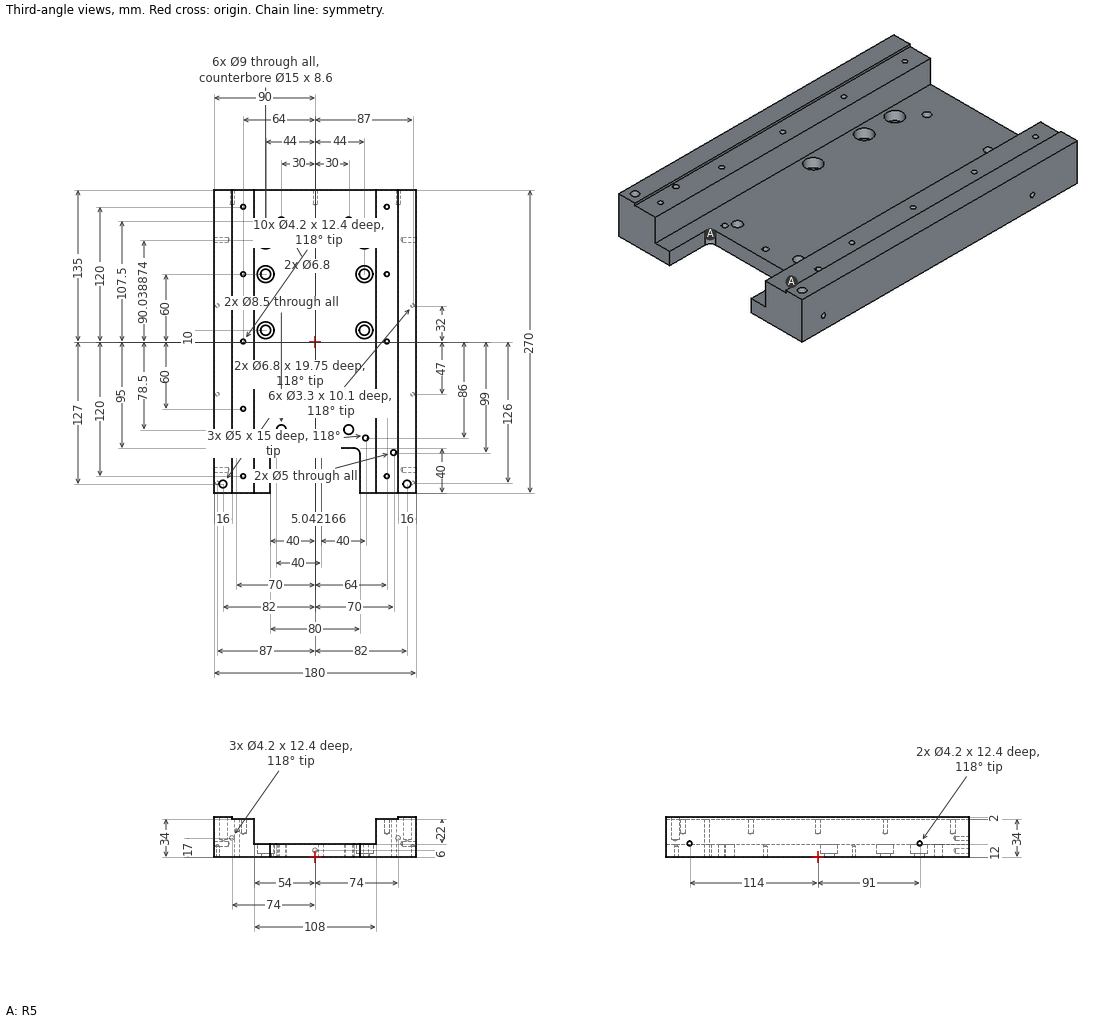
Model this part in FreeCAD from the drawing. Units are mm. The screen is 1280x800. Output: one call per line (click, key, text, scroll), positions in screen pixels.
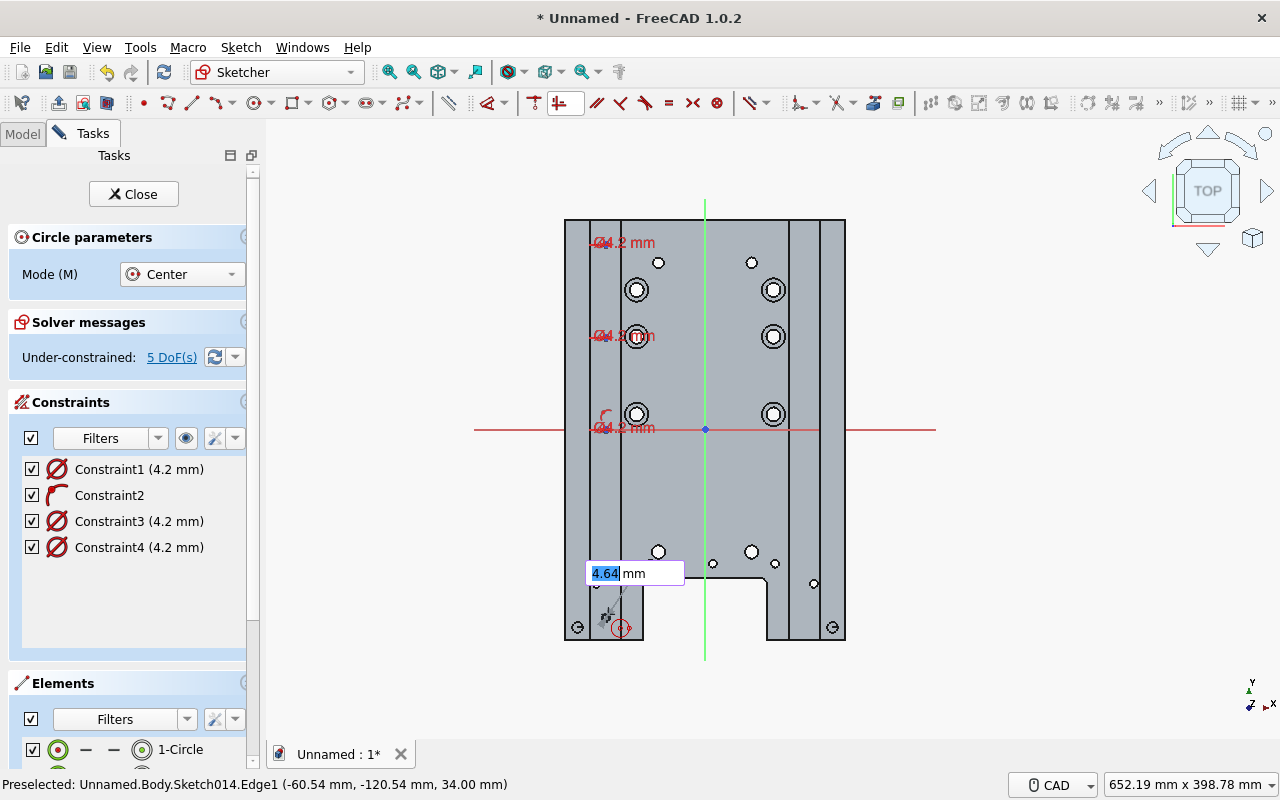
text(4.2)
key(Return)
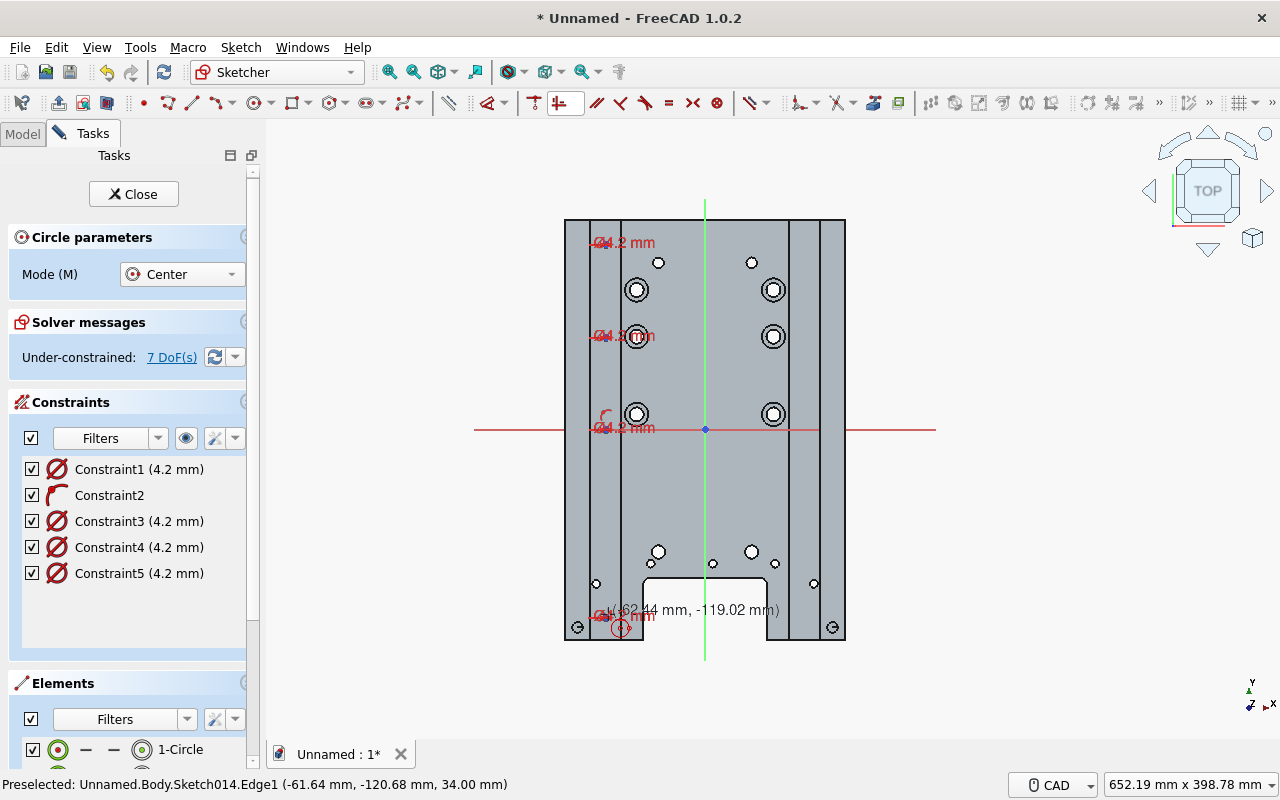
scroll(606, 523, up, 10)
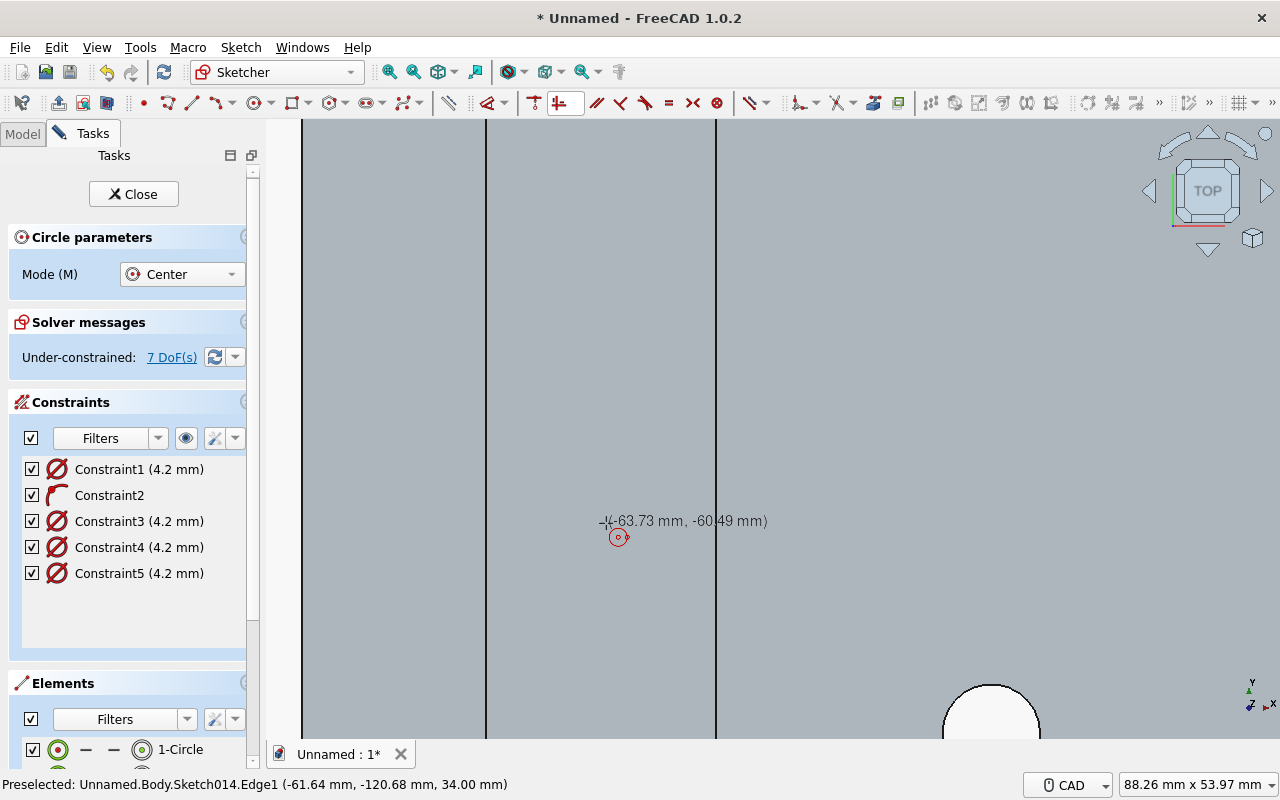
scroll(606, 523, down, 10)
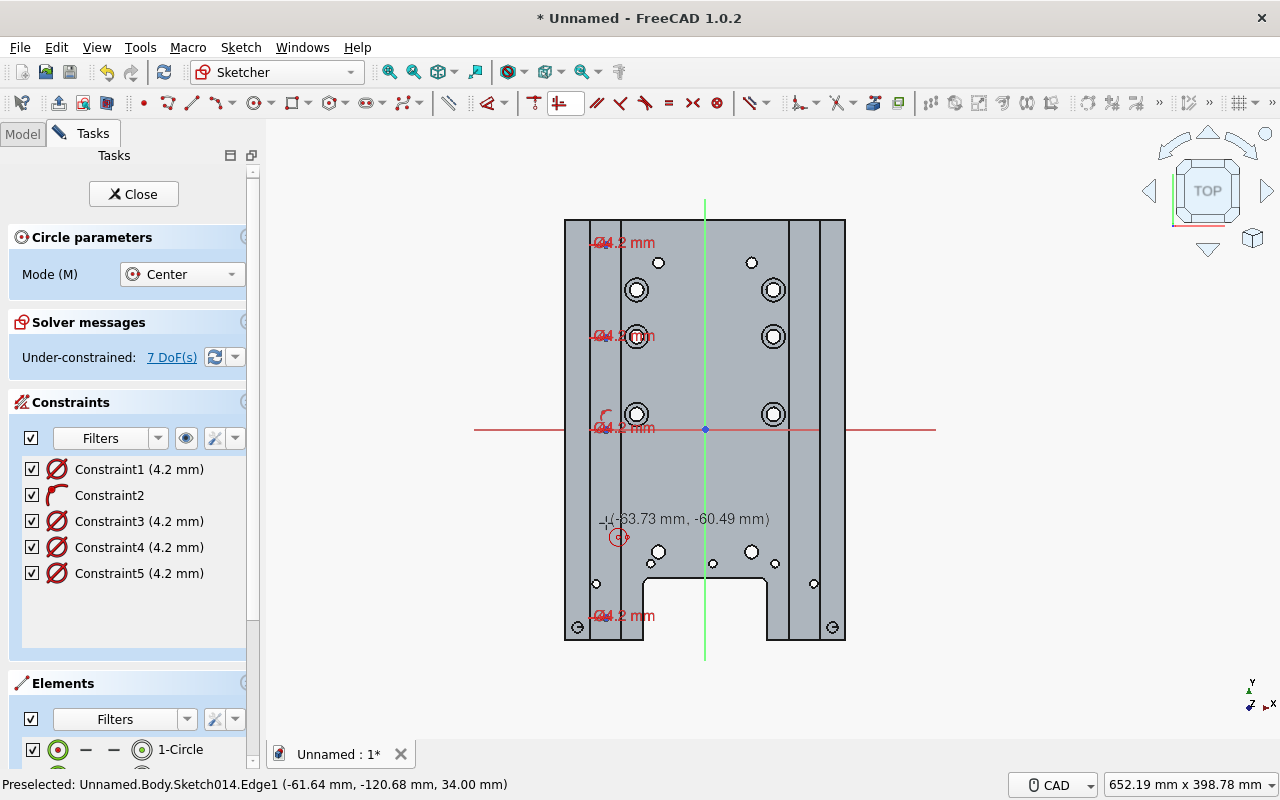
click(606, 523)
move(608, 521)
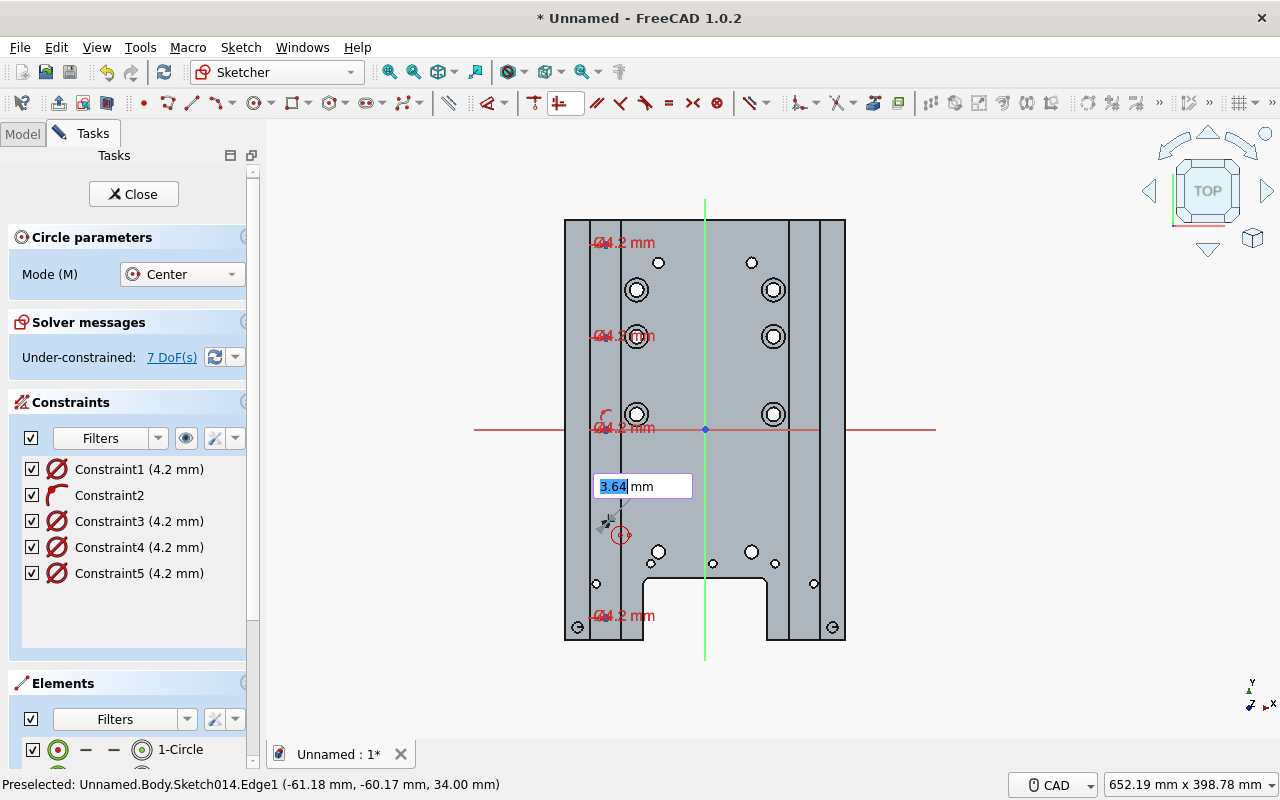
text(4.2)
key(Return)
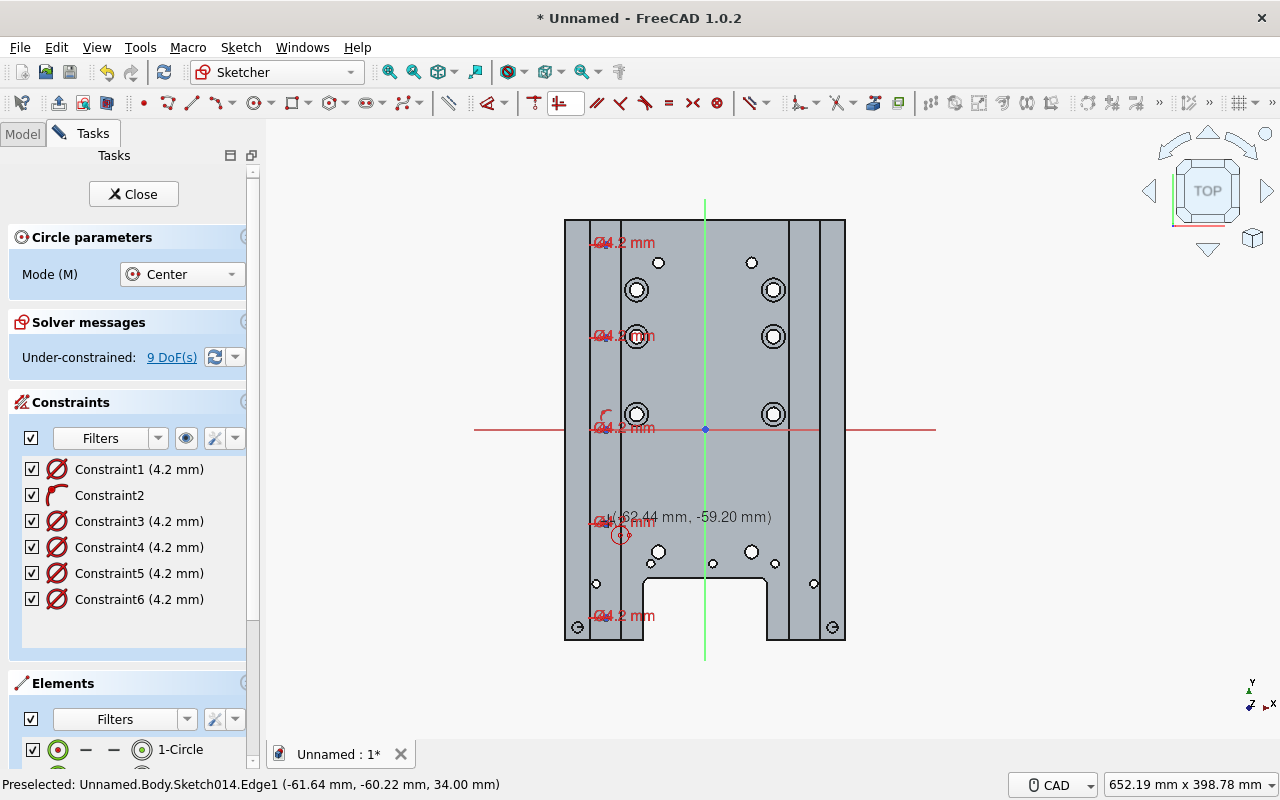
scroll(805, 523, up, 10)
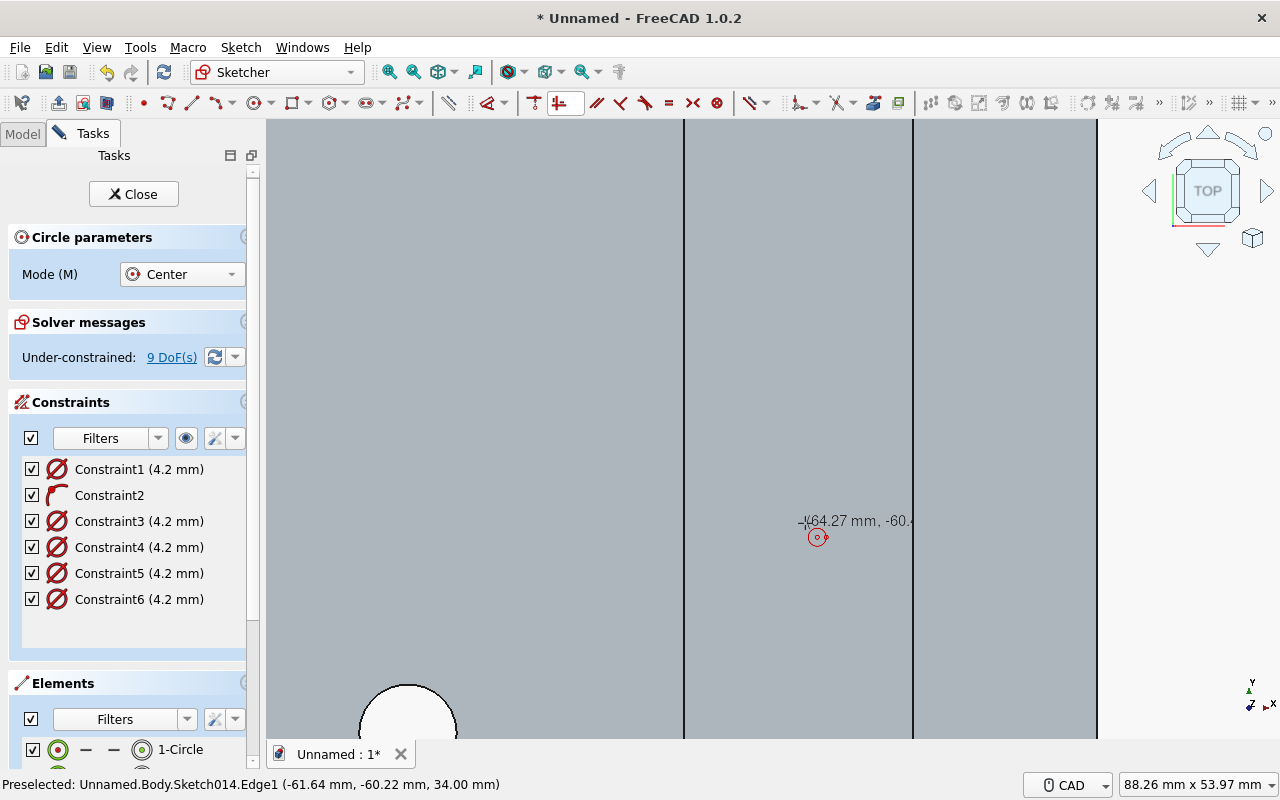
scroll(805, 523, down, 10)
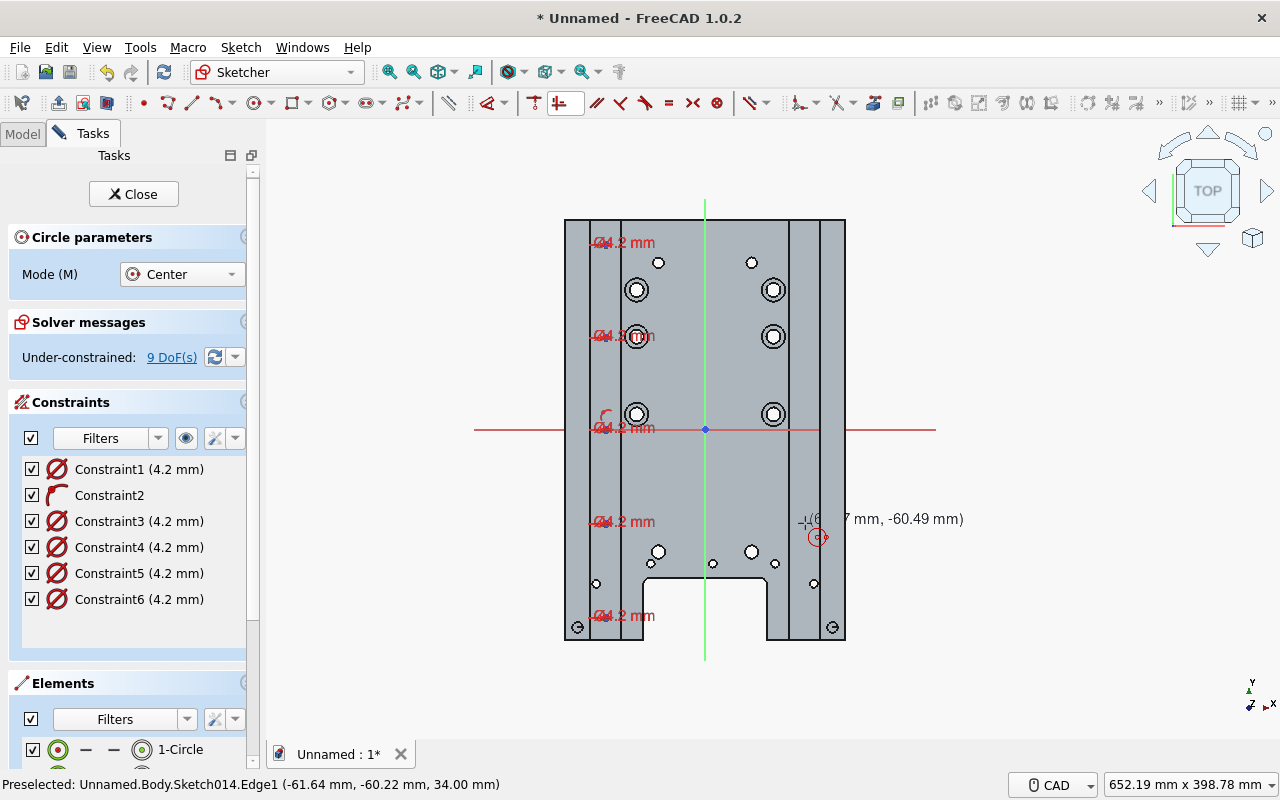
click(805, 523)
move(807, 521)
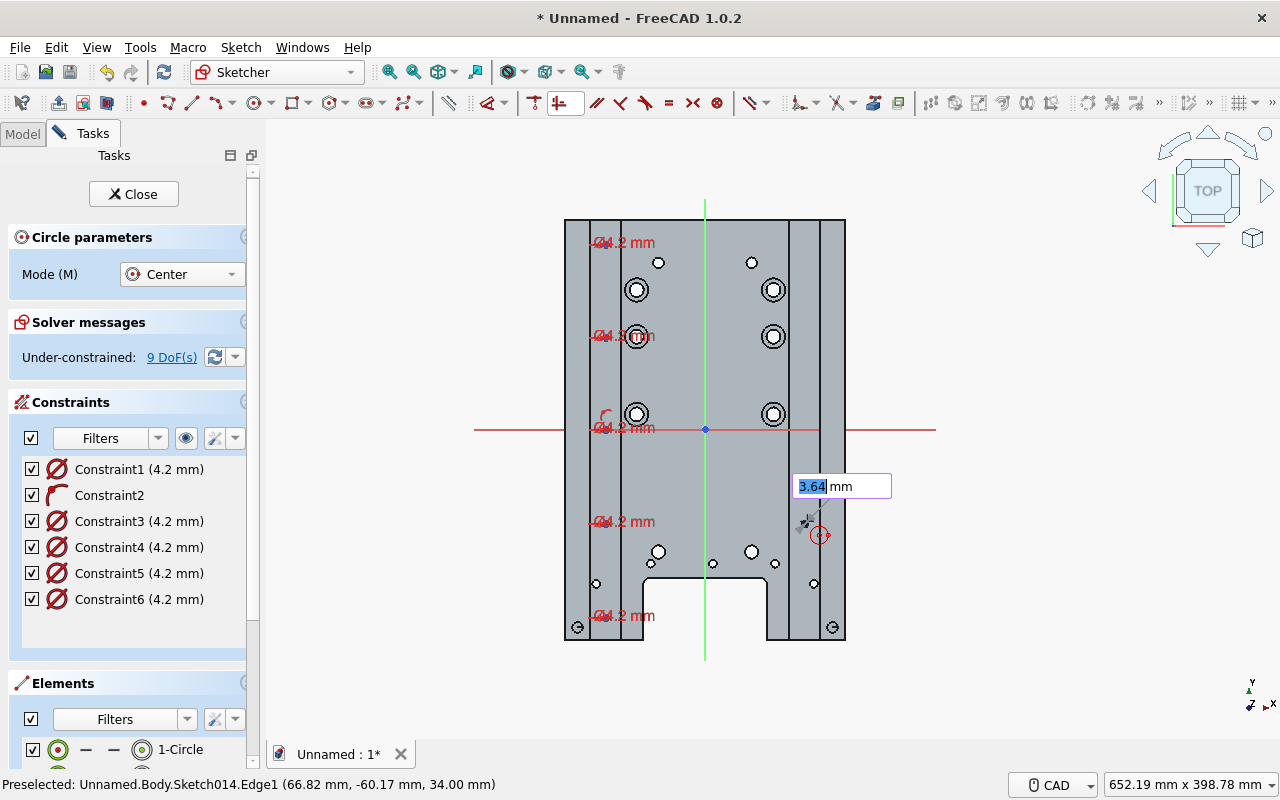
text(4.2)
key(Return)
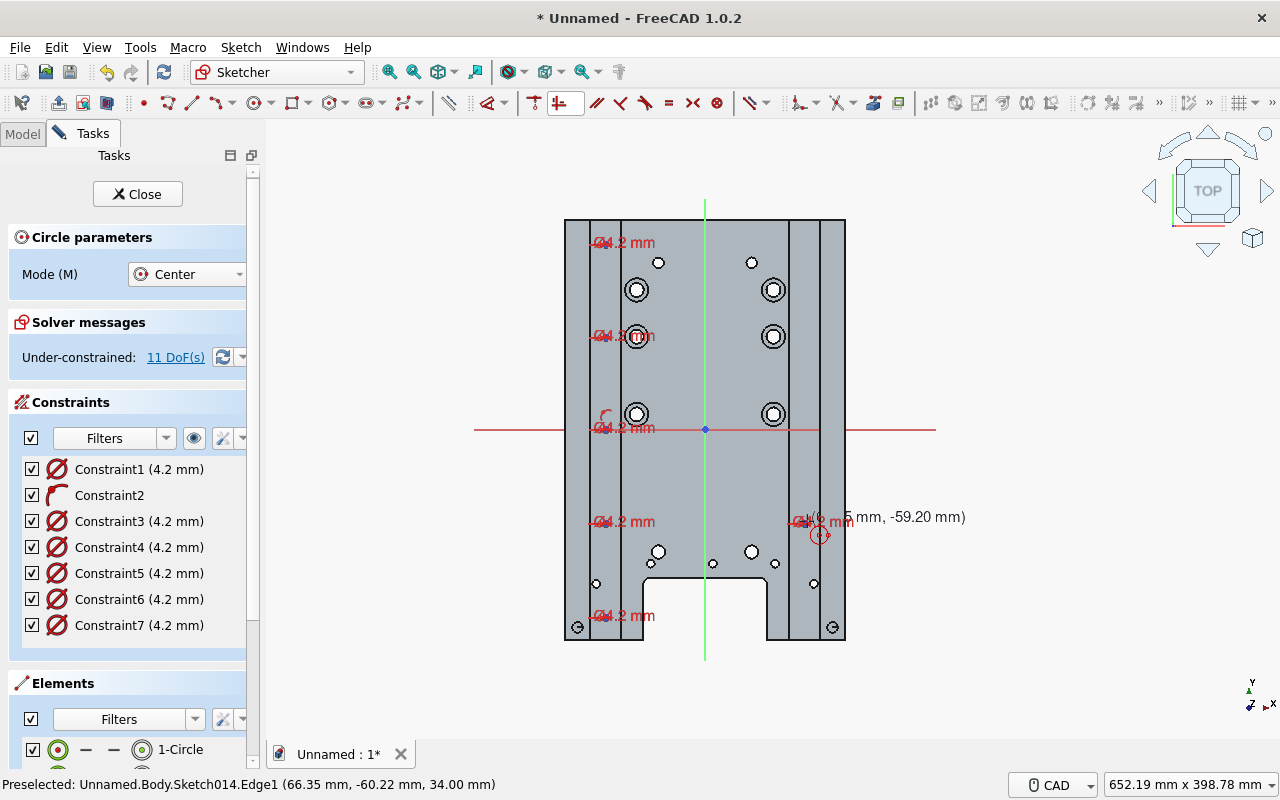
scroll(805, 617, up, 10)